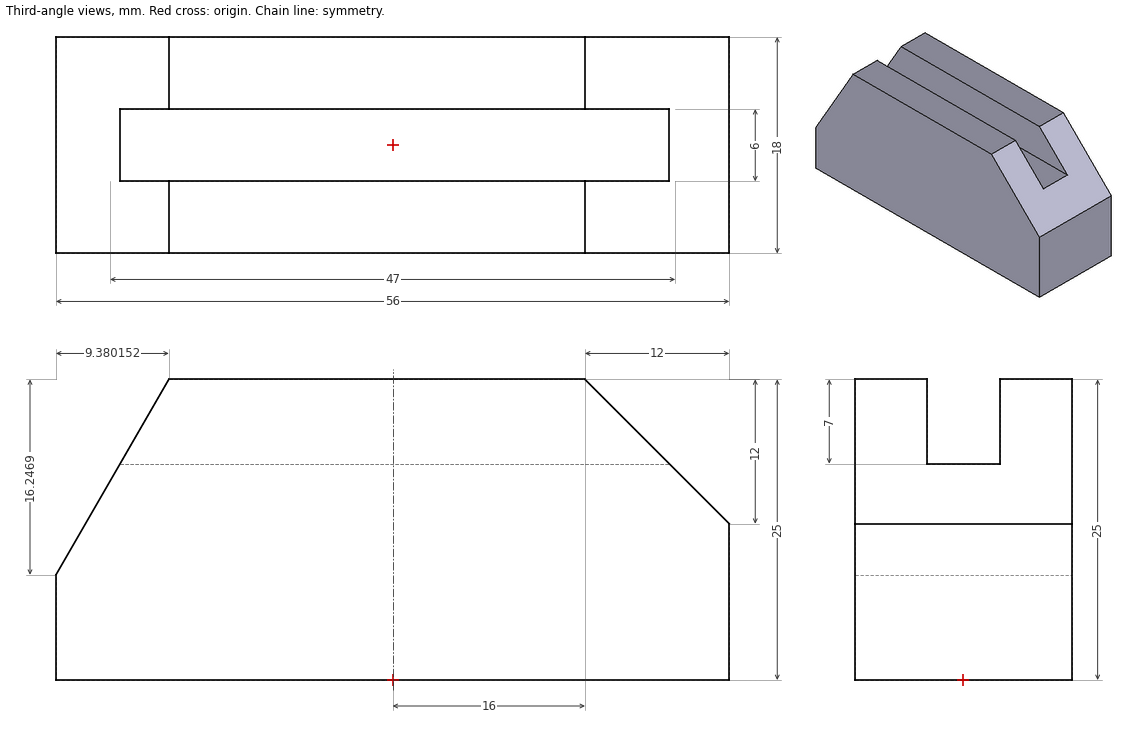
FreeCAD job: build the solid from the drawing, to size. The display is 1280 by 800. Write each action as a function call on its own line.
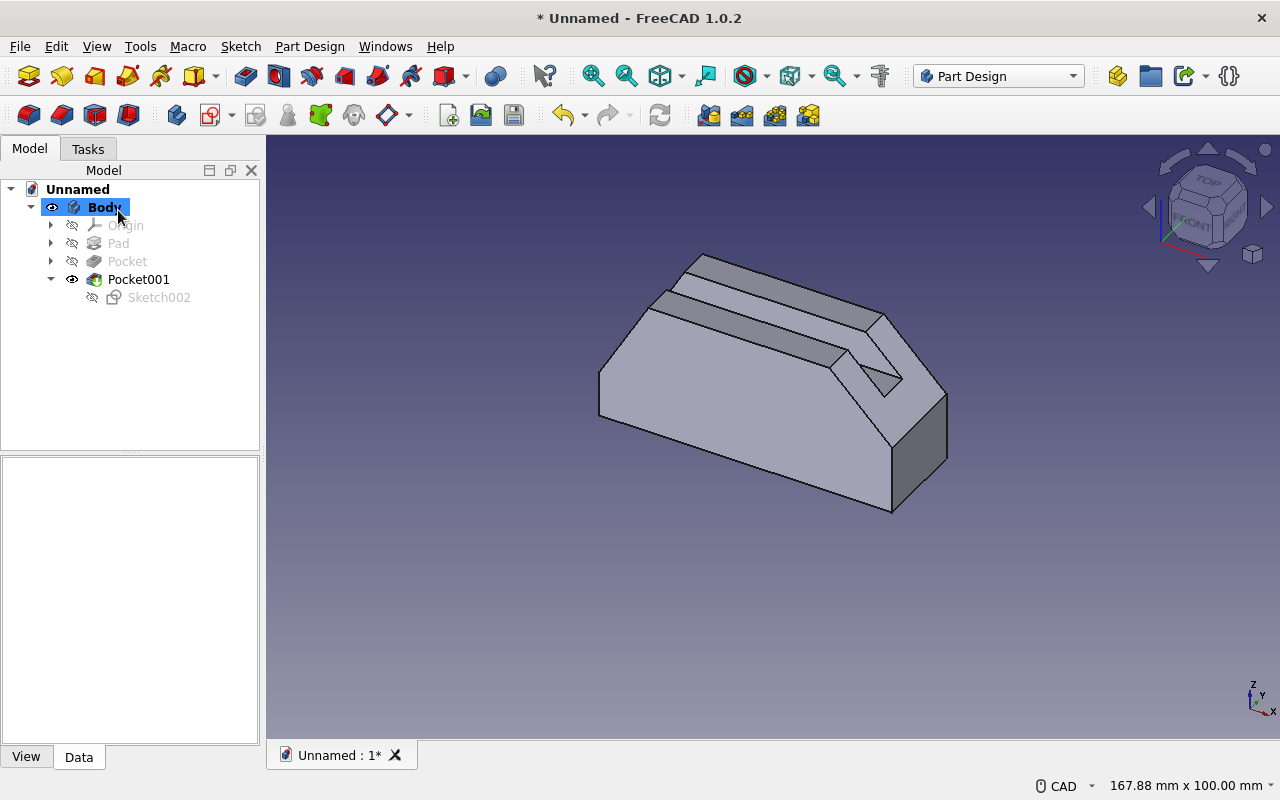
key(0)